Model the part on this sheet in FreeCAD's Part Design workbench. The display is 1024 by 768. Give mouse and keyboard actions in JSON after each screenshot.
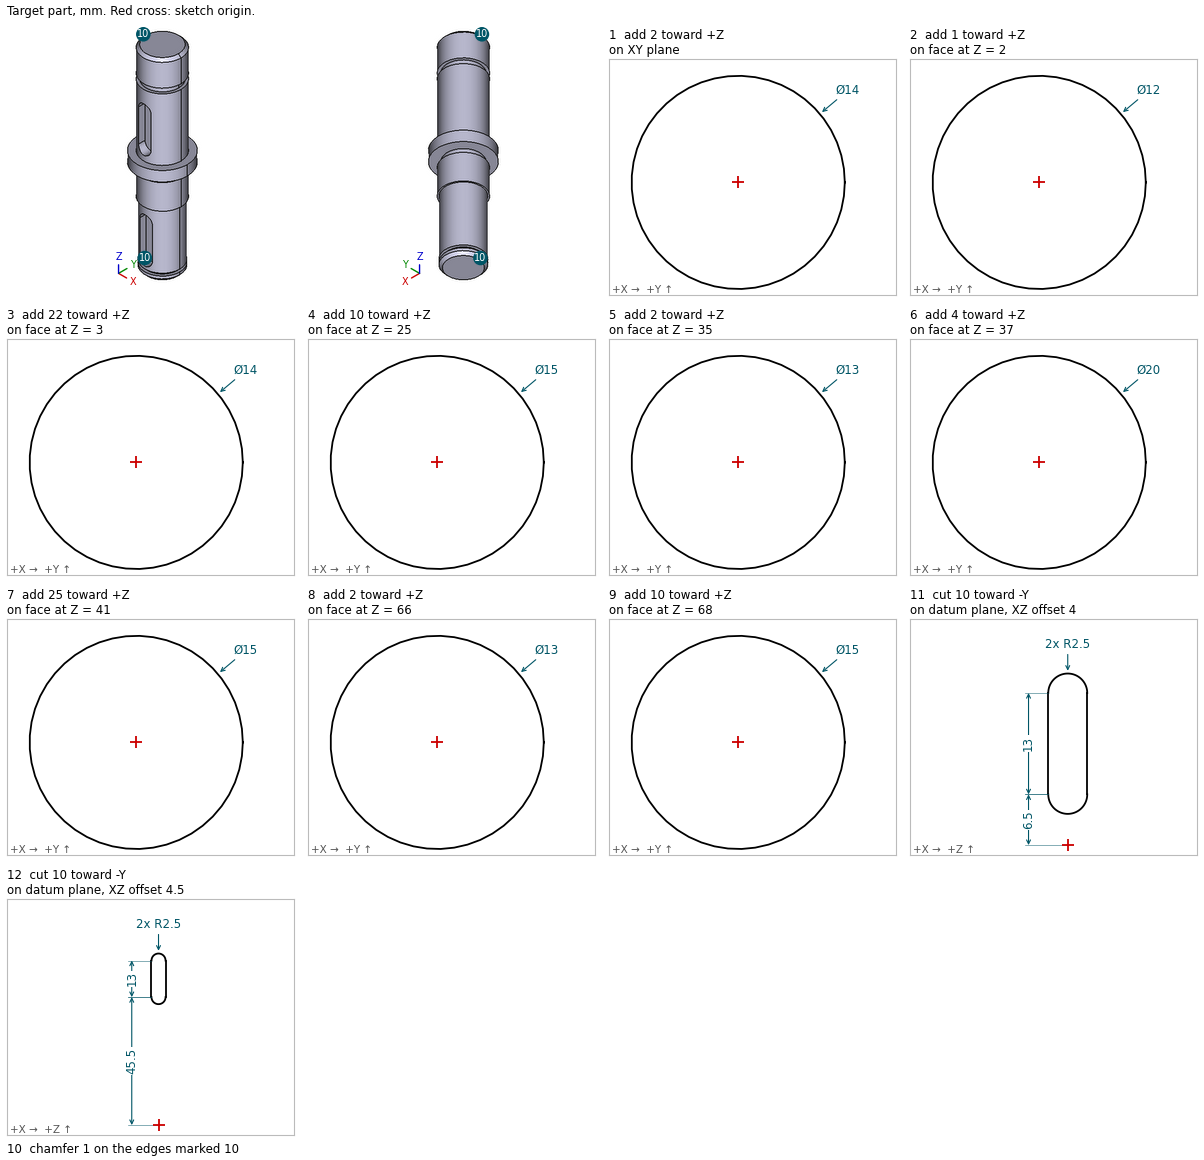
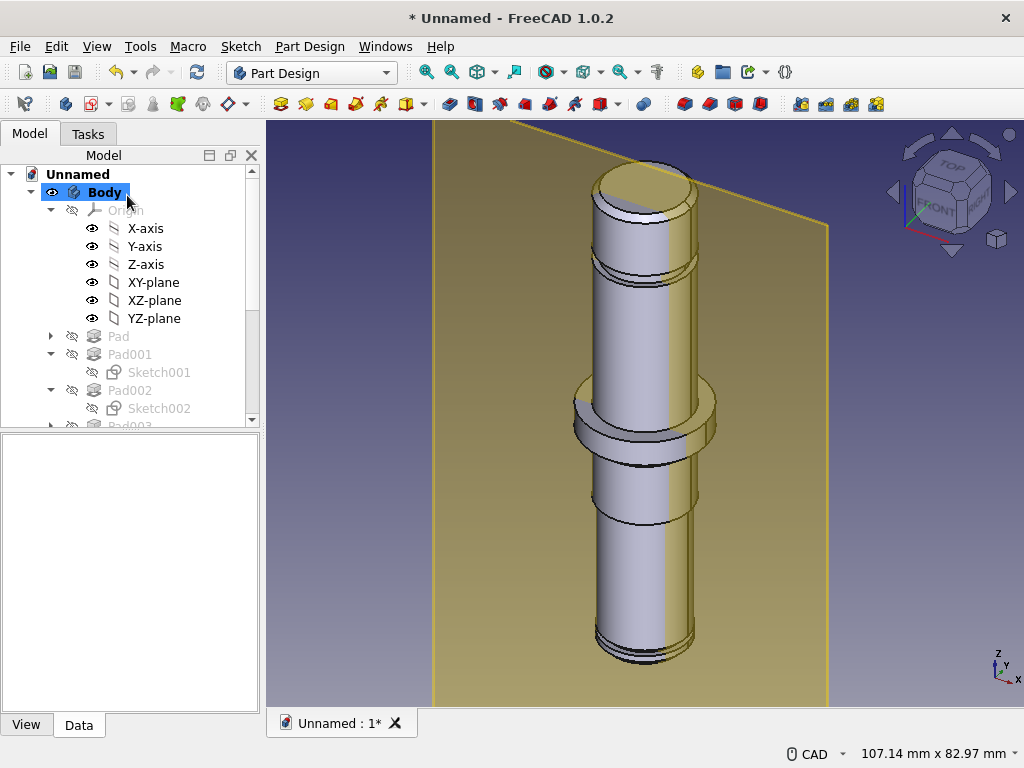
{"action": "scroll", "coordinate": [101, 296], "scroll_direction": "down", "scroll_amount": 3}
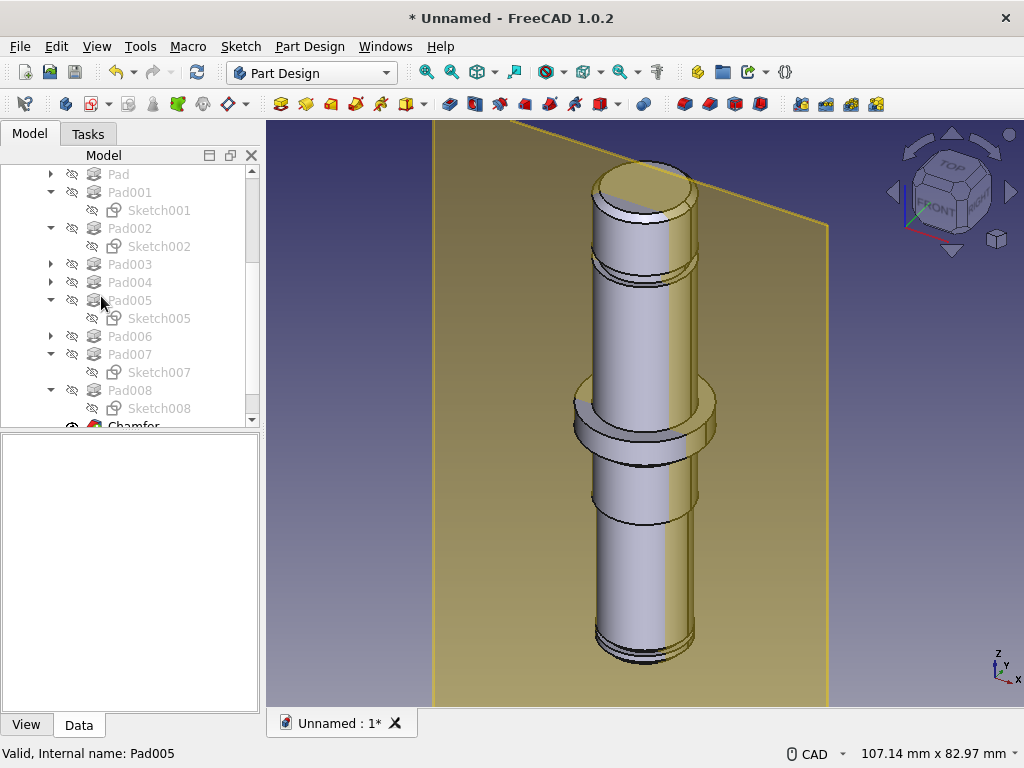
{"action": "scroll", "coordinate": [141, 296], "scroll_direction": "up", "scroll_amount": 15}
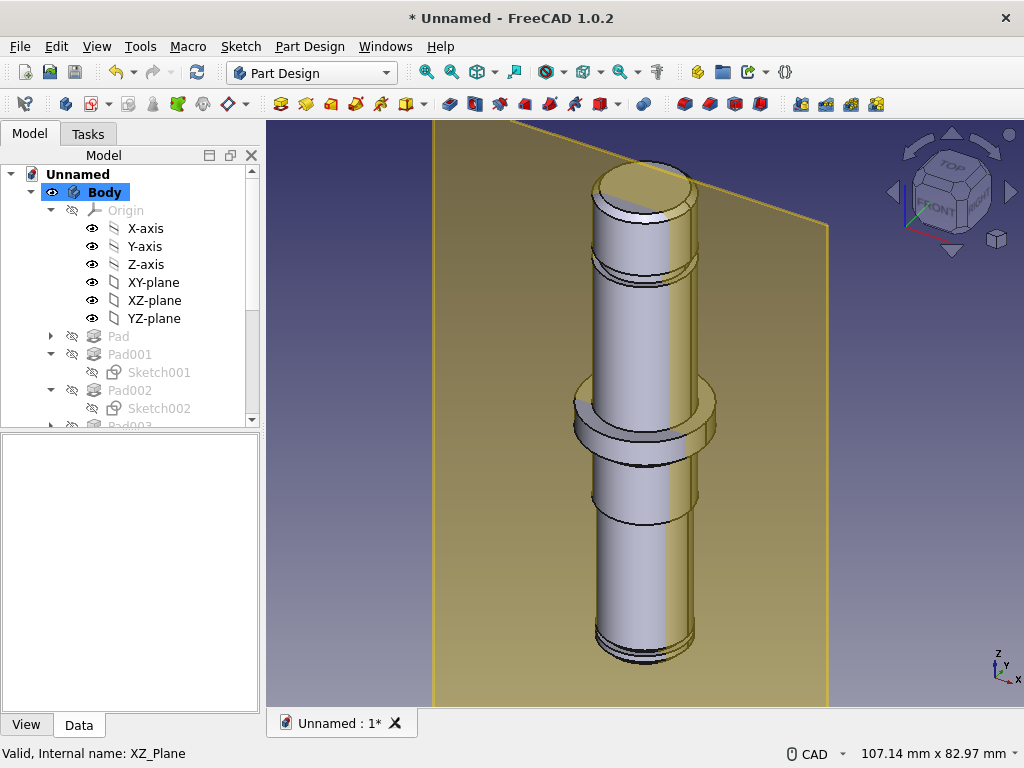
{"action": "scroll", "coordinate": [101, 296], "scroll_direction": "down", "scroll_amount": 6}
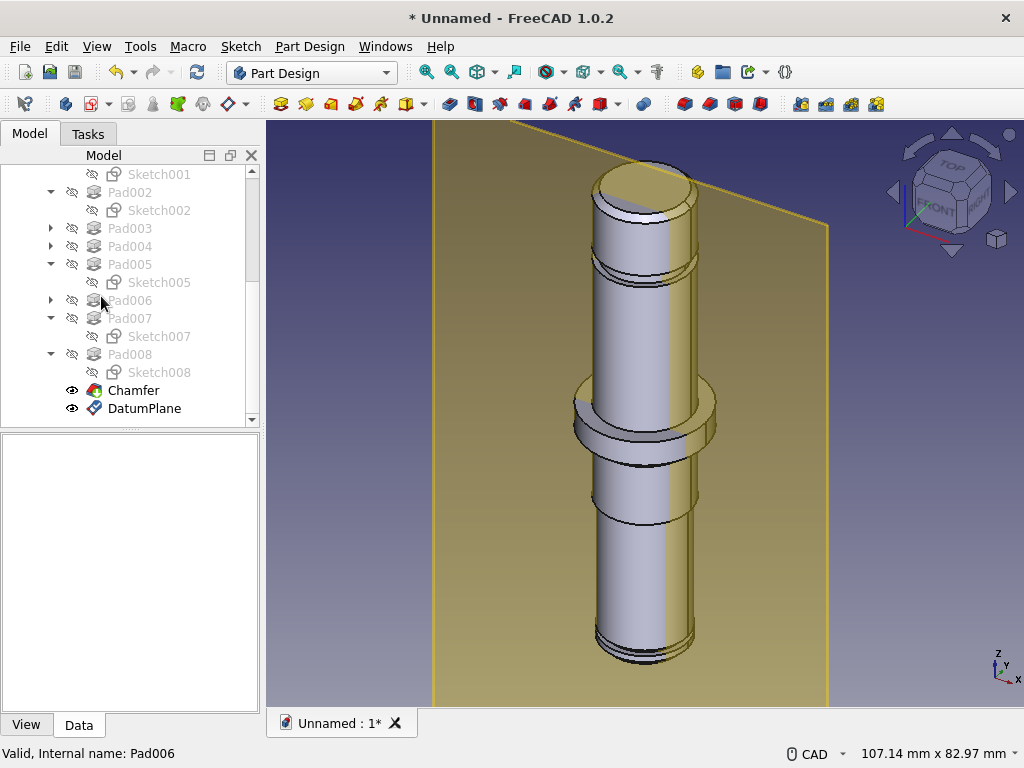
{"action": "left_click", "coordinate": [117, 408]}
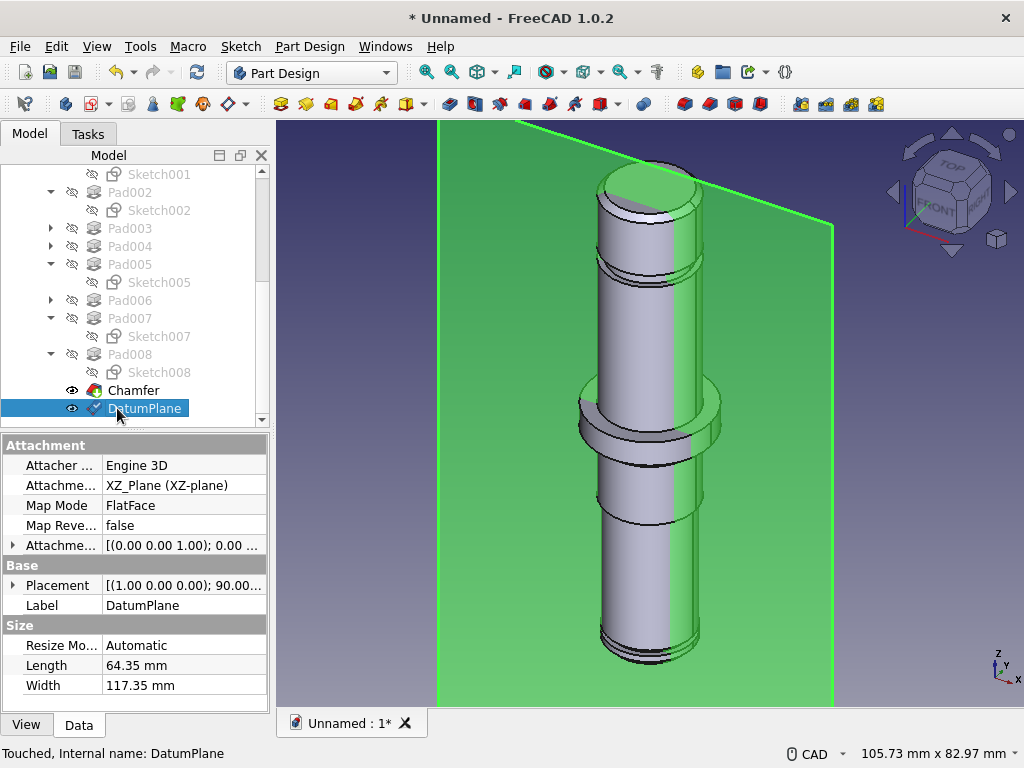
{"action": "left_click", "coordinate": [90, 104]}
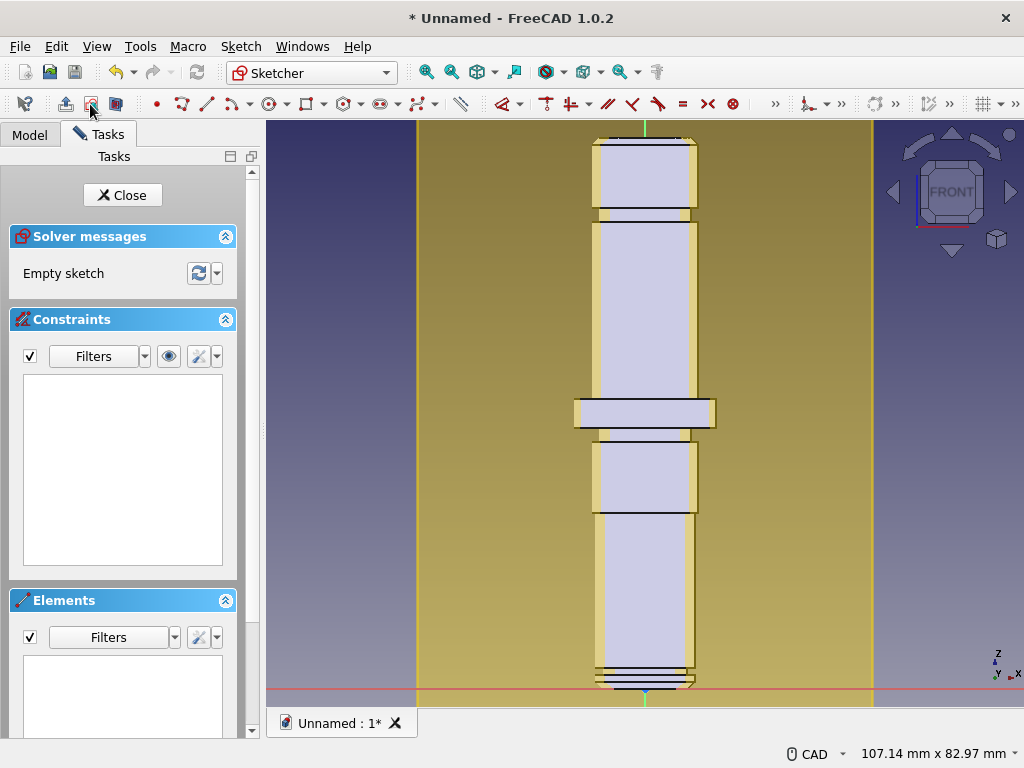
{"action": "left_click", "coordinate": [116, 104]}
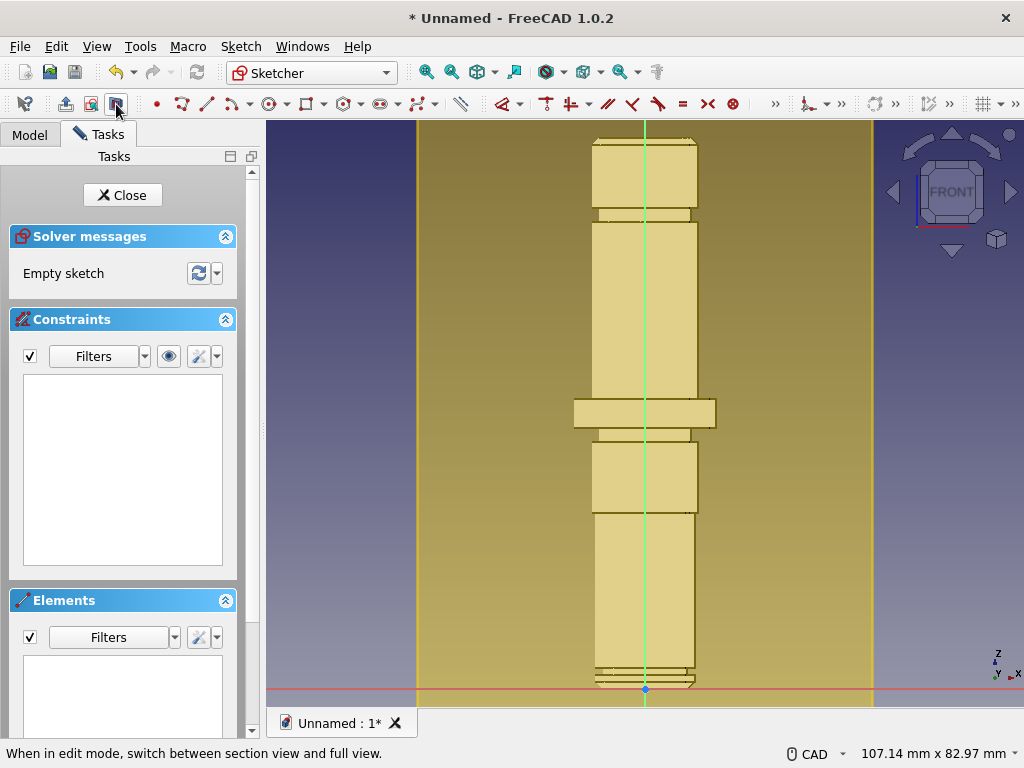
{"action": "scroll", "coordinate": [576, 414], "scroll_direction": "down", "scroll_amount": 5}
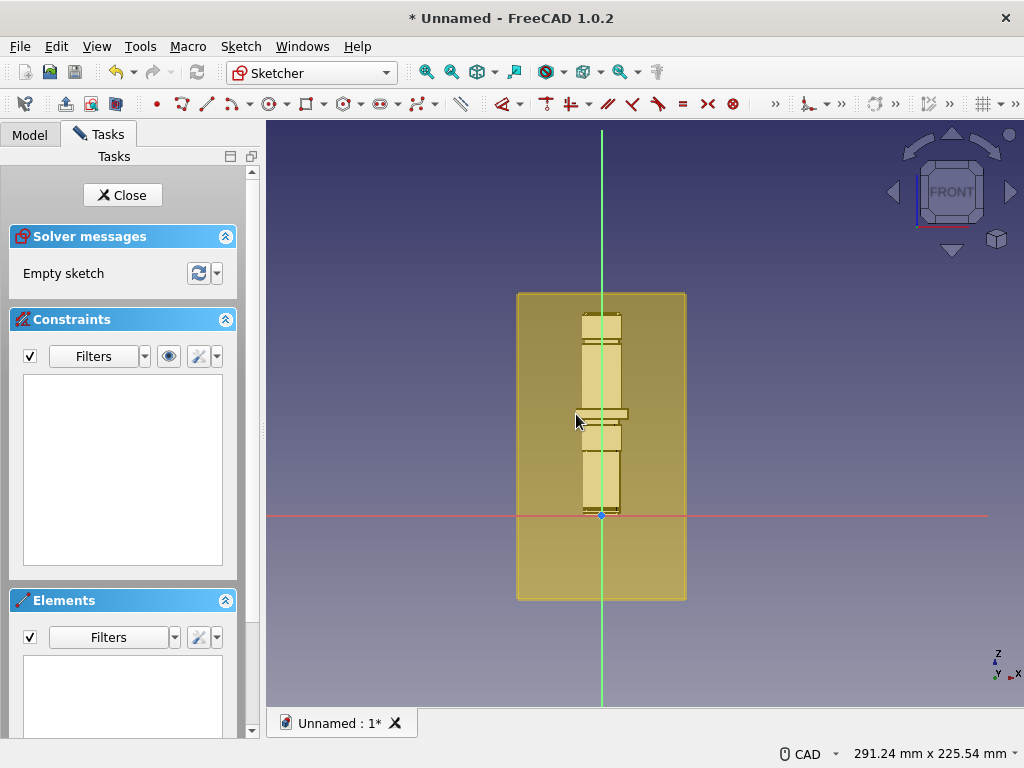
{"action": "scroll", "coordinate": [607, 502], "scroll_direction": "up", "scroll_amount": 9}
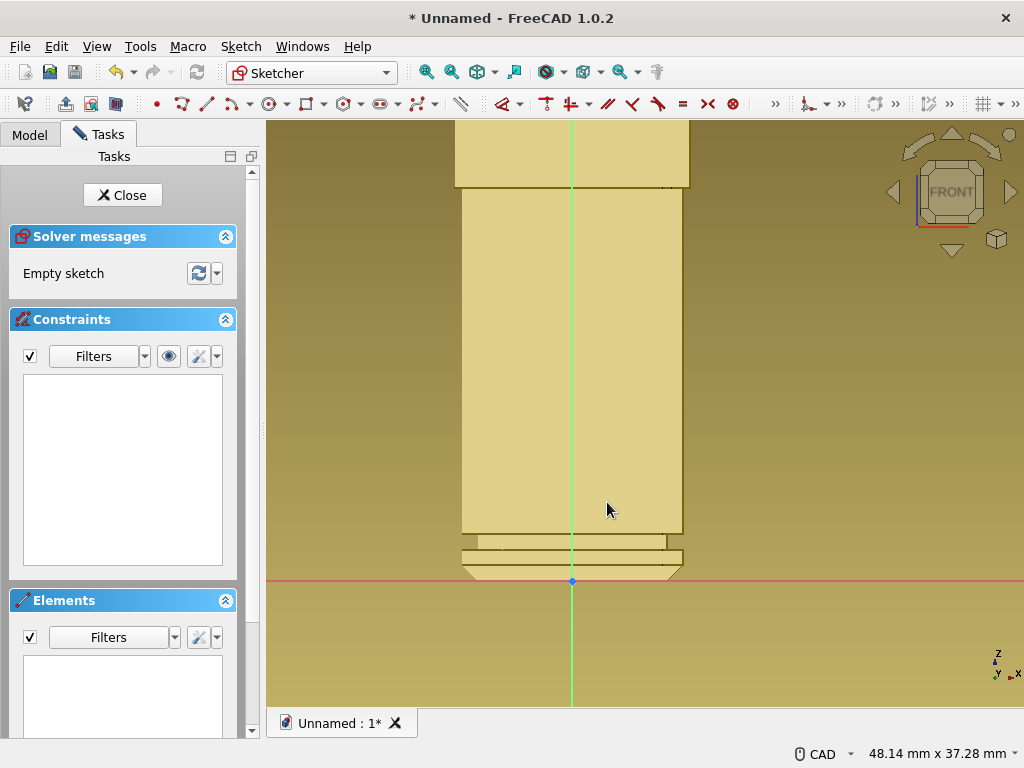
{"action": "left_click", "coordinate": [380, 104]}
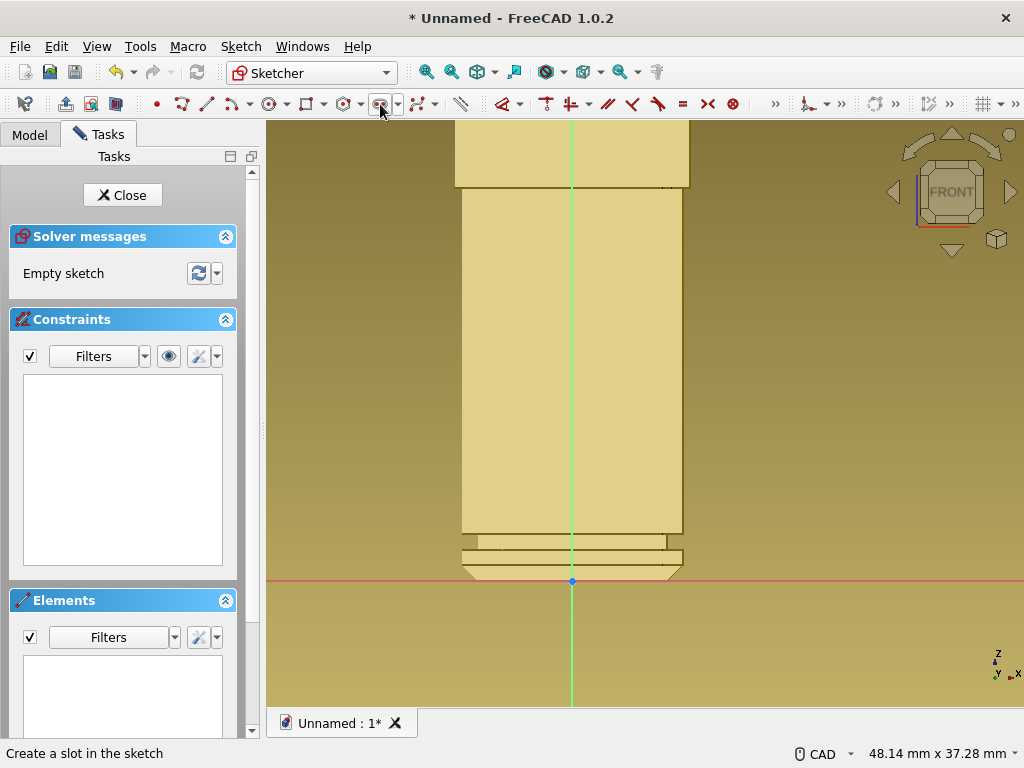
{"action": "left_click", "coordinate": [572, 479]}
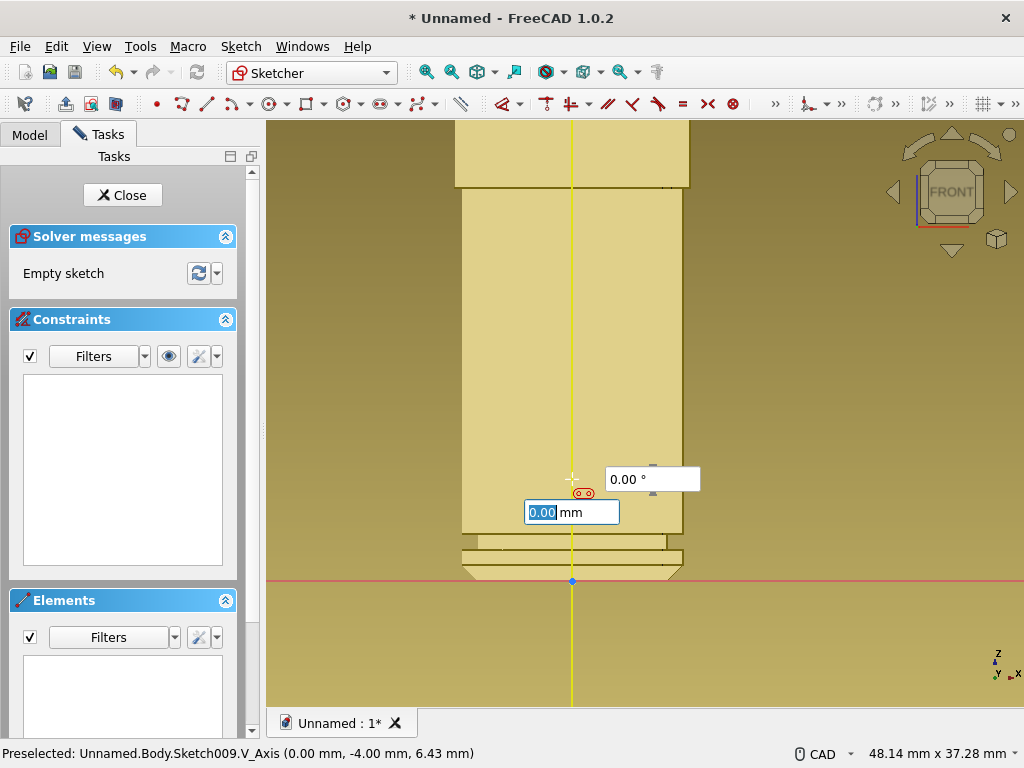
{"action": "left_click", "coordinate": [581, 274]}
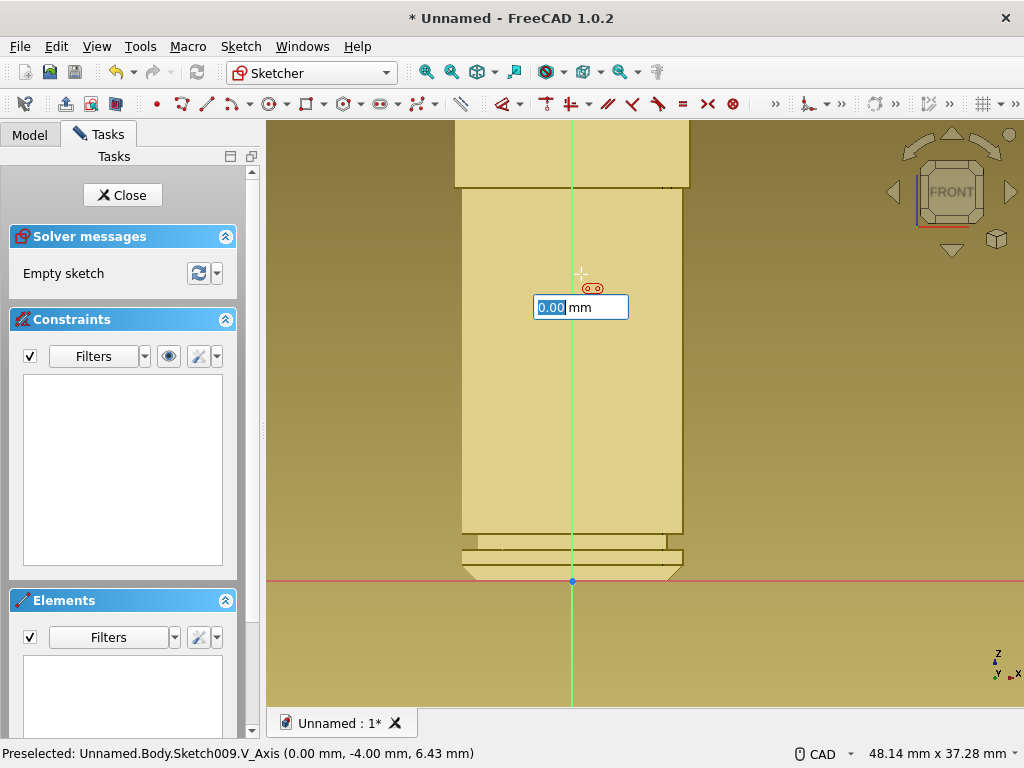
{"action": "left_click", "coordinate": [533, 377]}
{"action": "key", "text": "Escape"}